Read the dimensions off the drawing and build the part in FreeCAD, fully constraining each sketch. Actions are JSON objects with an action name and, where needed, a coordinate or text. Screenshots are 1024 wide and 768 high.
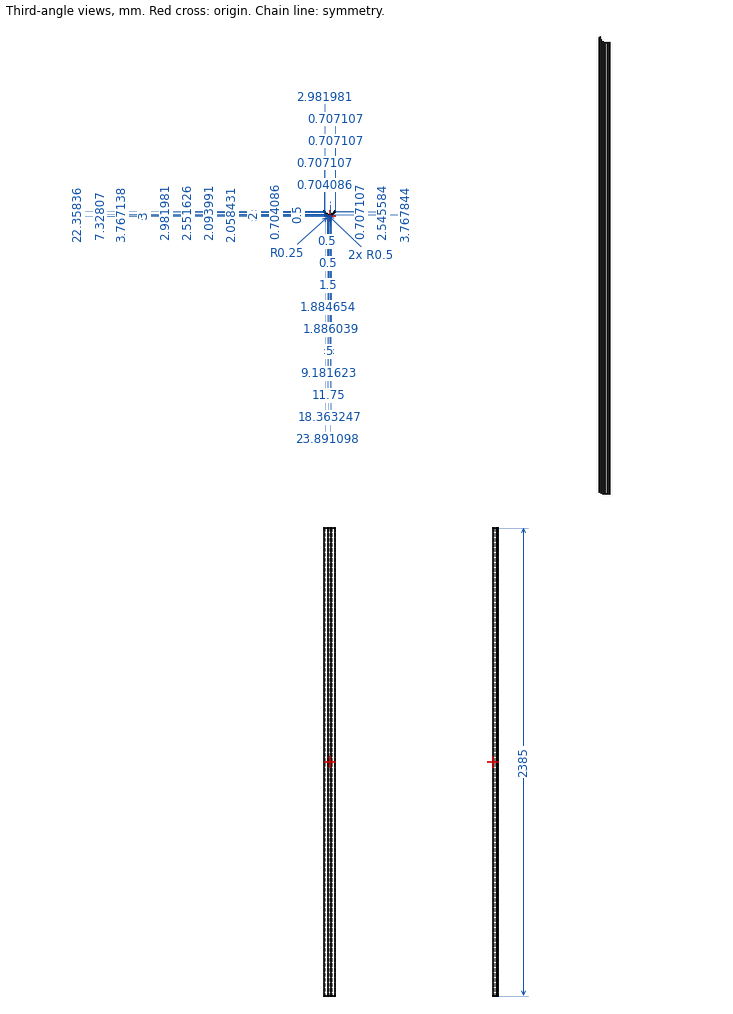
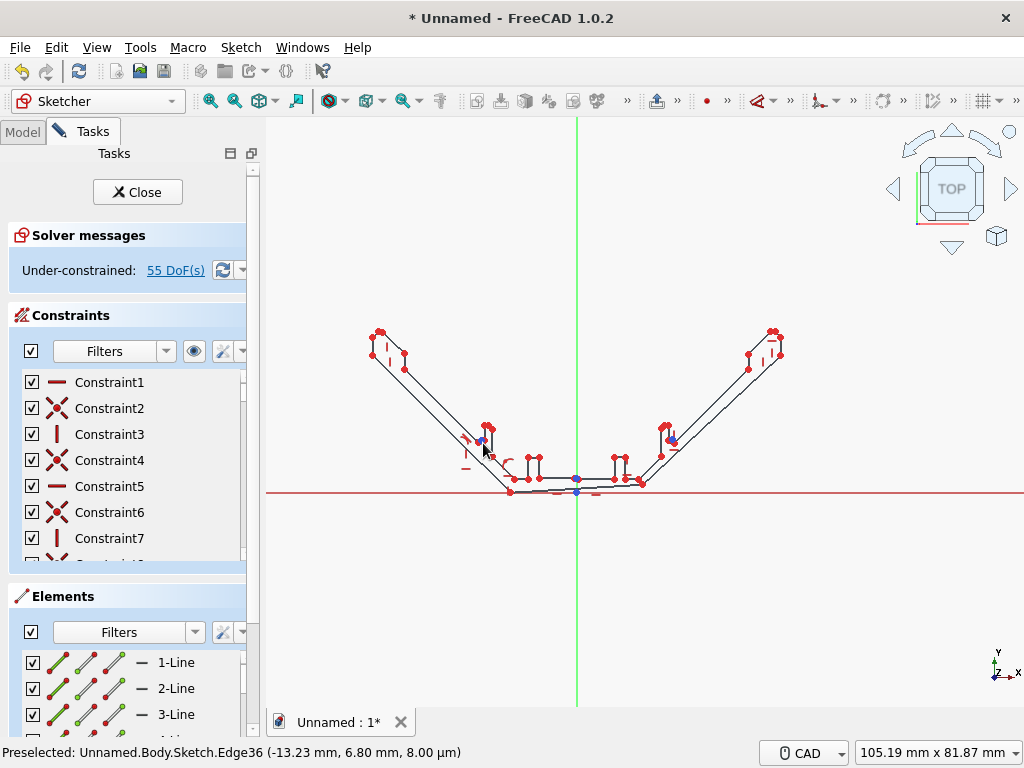
{"action": "scroll", "coordinate": [727, 391], "scroll_direction": "up", "scroll_amount": 2}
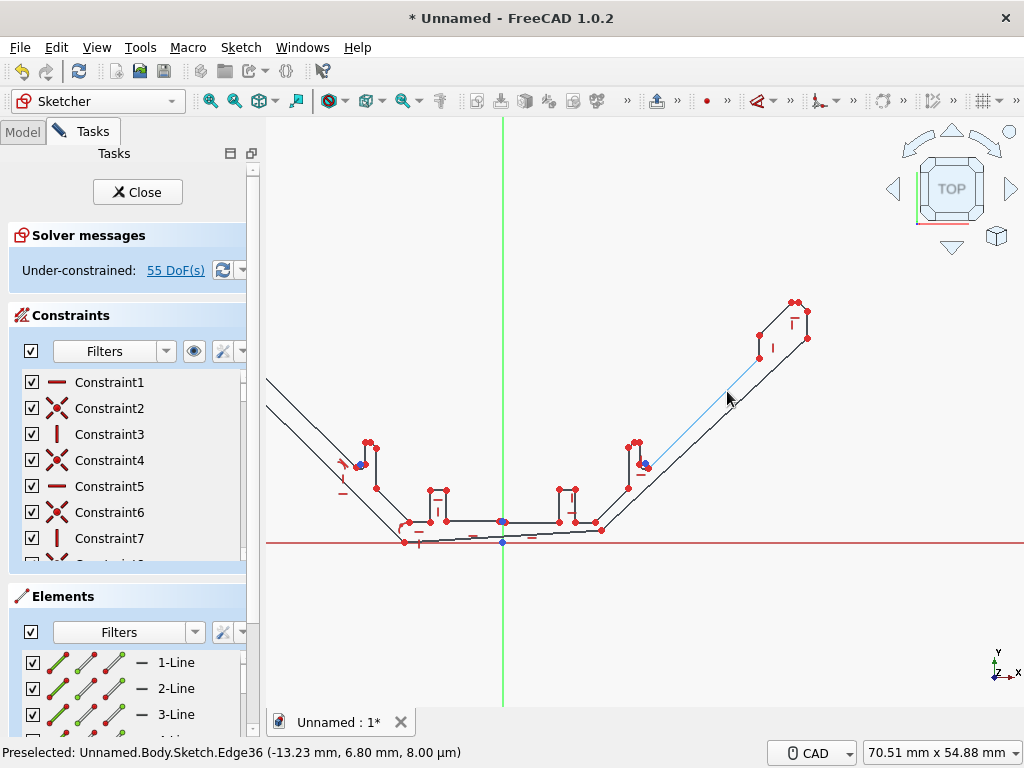
{"action": "left_click", "coordinate": [726, 391]}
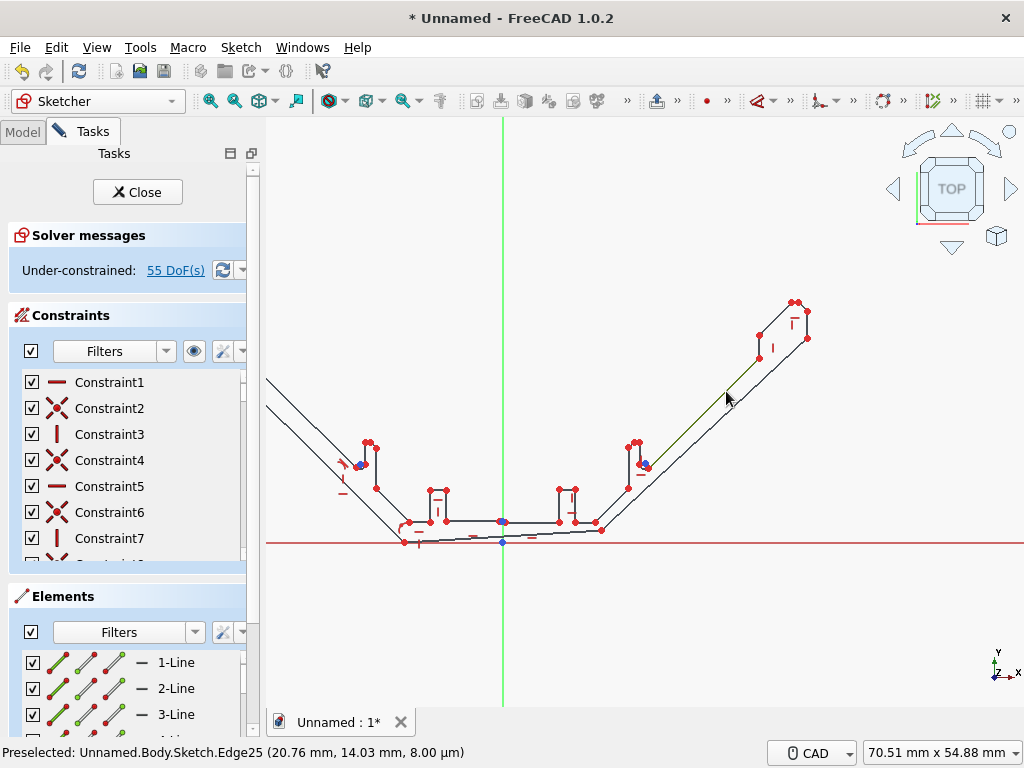
{"action": "scroll", "coordinate": [643, 469], "scroll_direction": "up", "scroll_amount": 5}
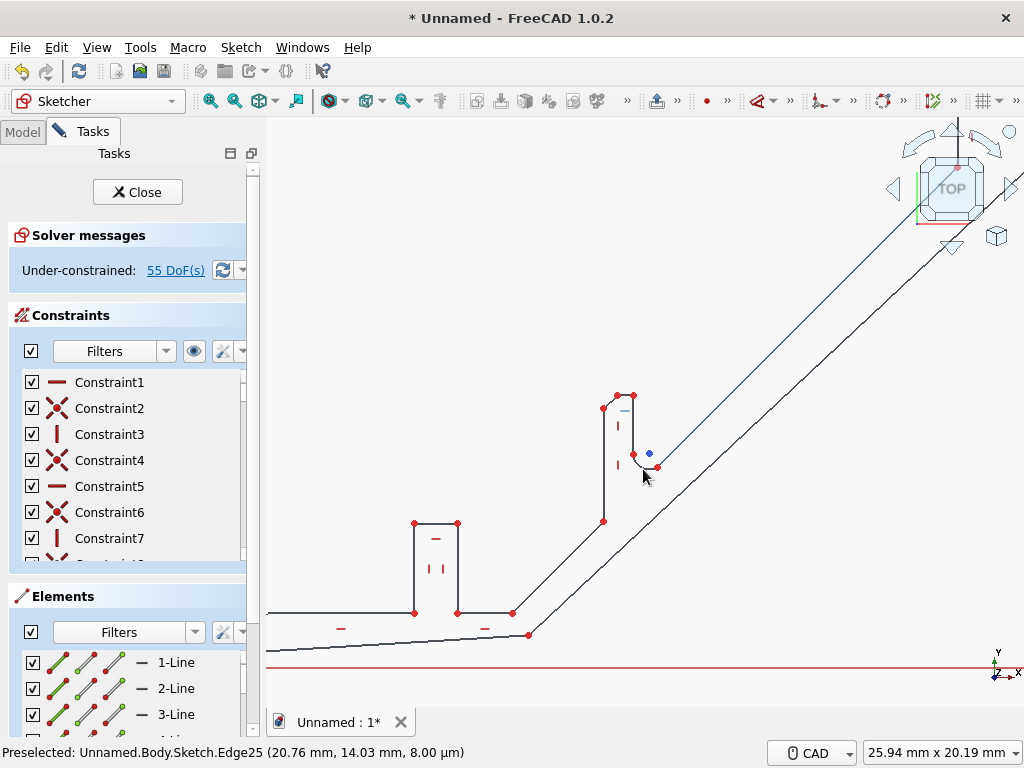
{"action": "left_click", "coordinate": [642, 468]}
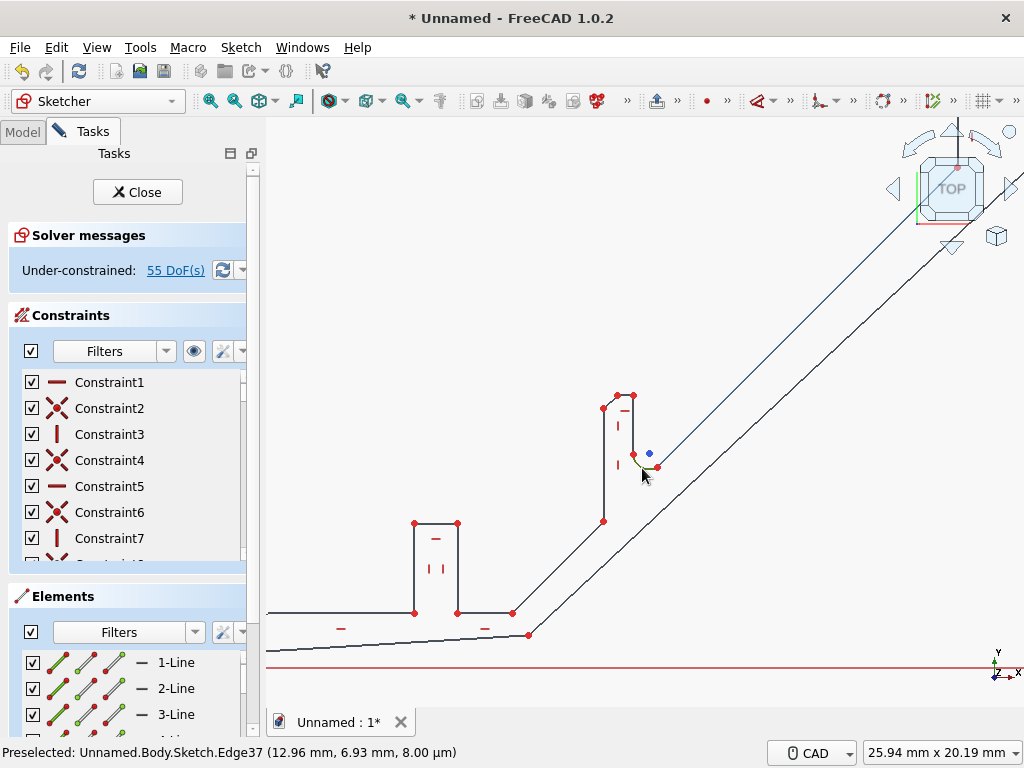
{"action": "key", "text": "t"}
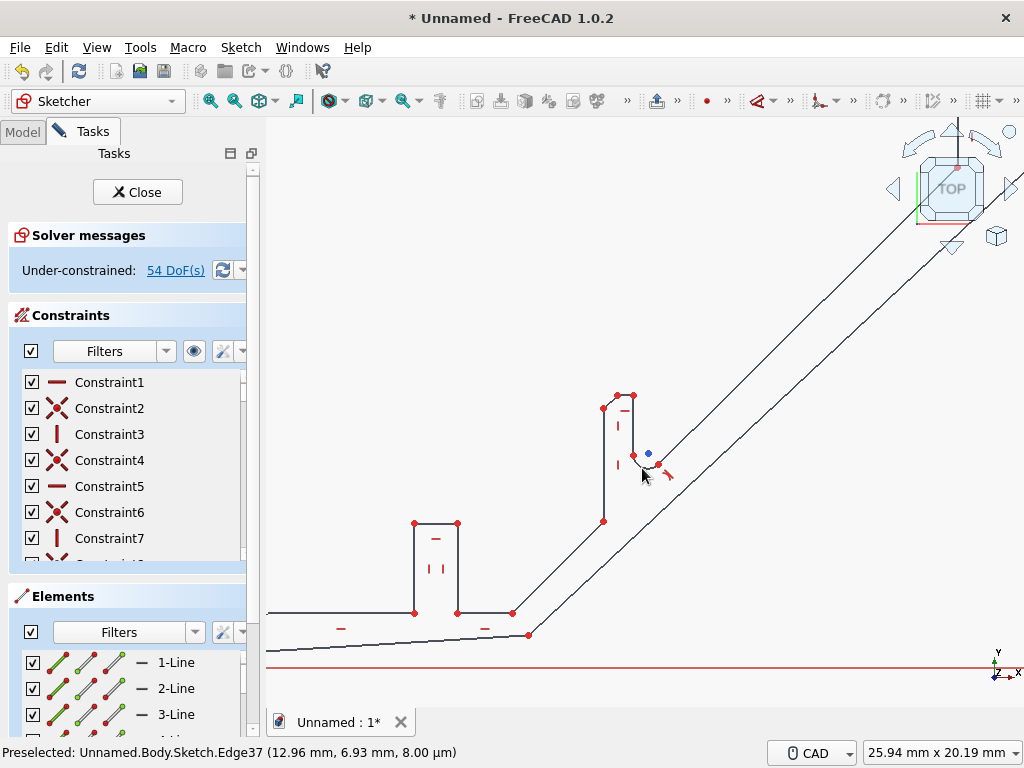
{"action": "left_click", "coordinate": [633, 437]}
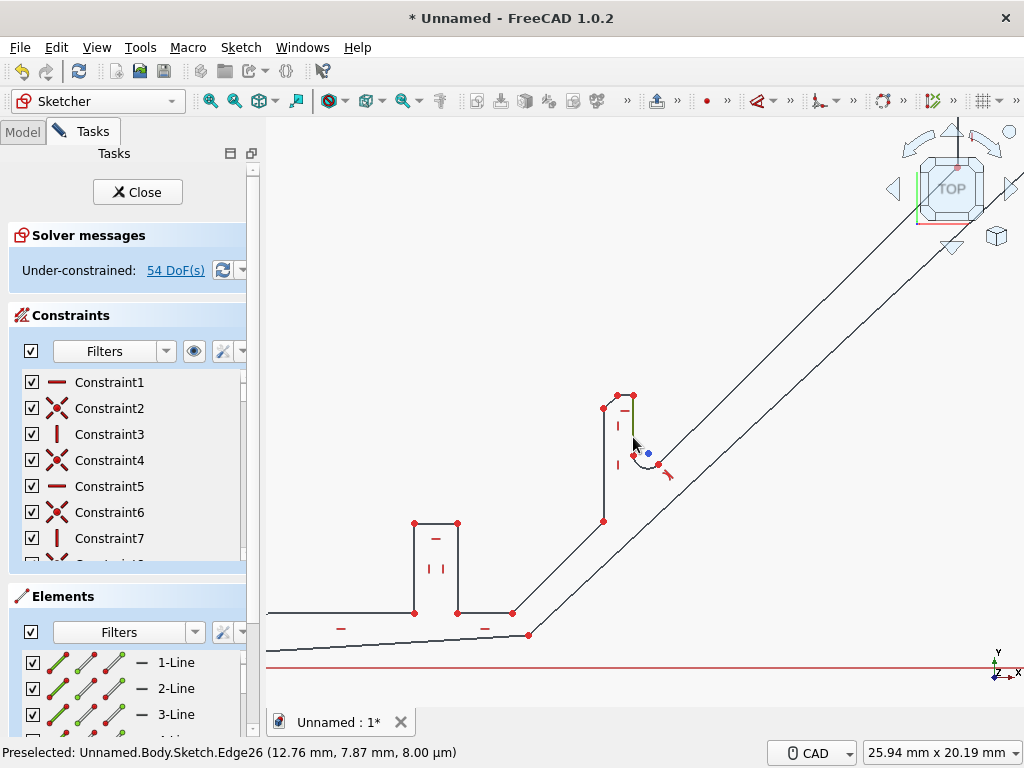
{"action": "scroll", "coordinate": [638, 464], "scroll_direction": "up", "scroll_amount": 2}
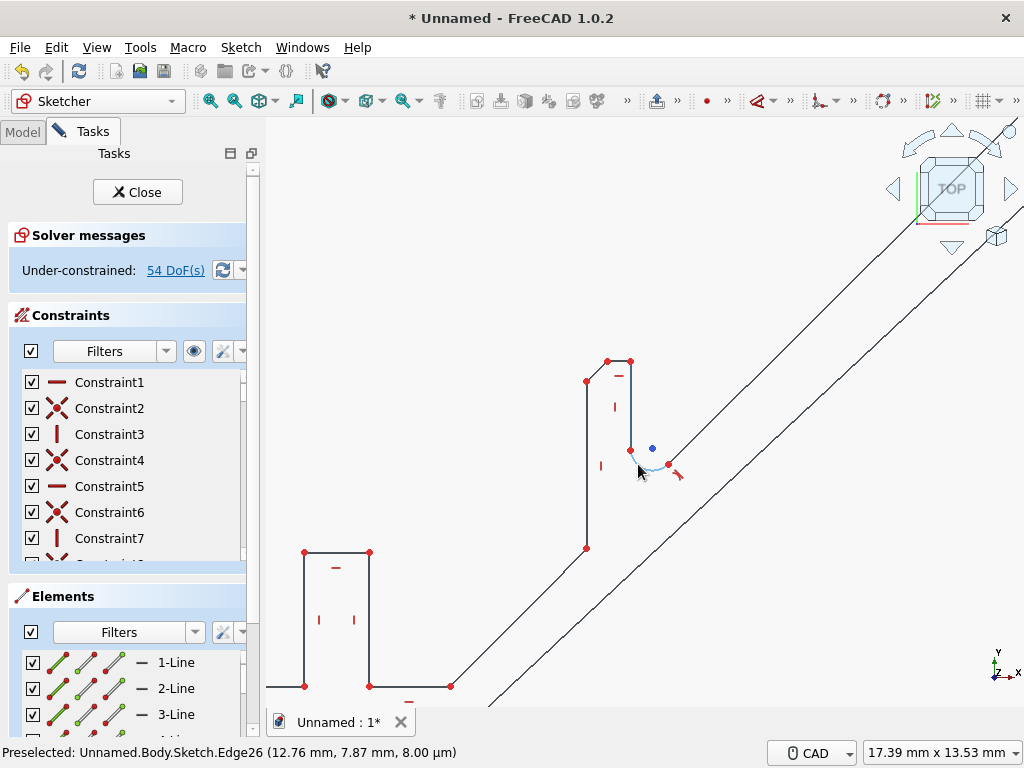
{"action": "left_click", "coordinate": [637, 464]}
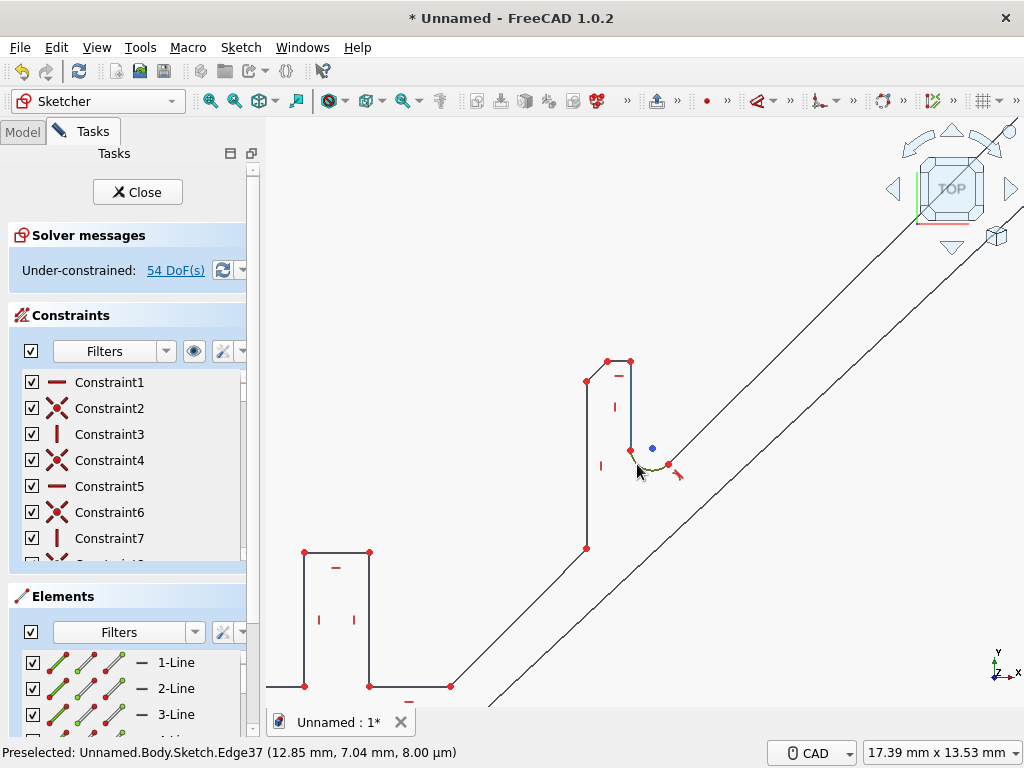
{"action": "key", "text": "t"}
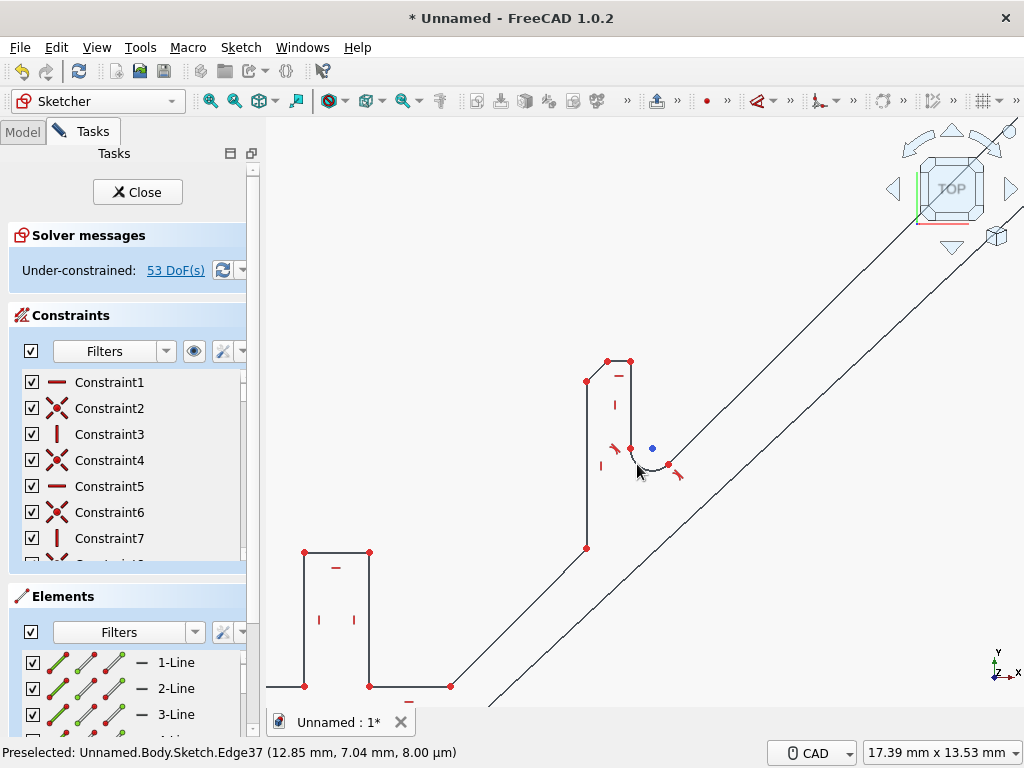
{"action": "scroll", "coordinate": [676, 438], "scroll_direction": "down", "scroll_amount": 9}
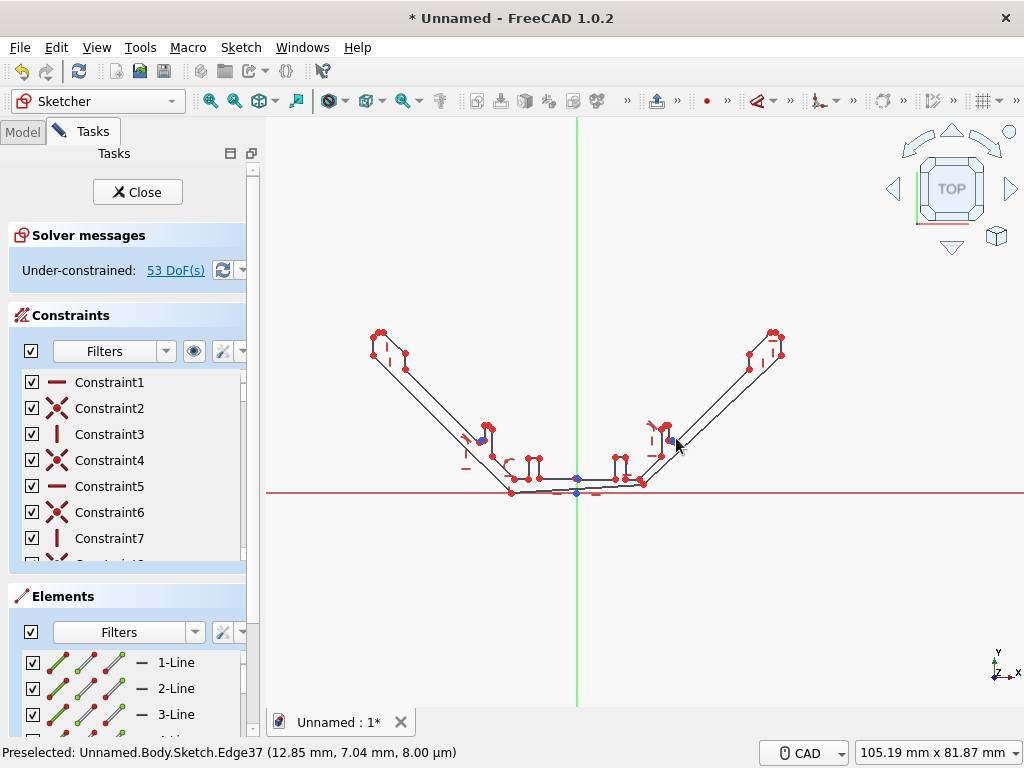
{"action": "scroll", "coordinate": [381, 333], "scroll_direction": "up", "scroll_amount": 10}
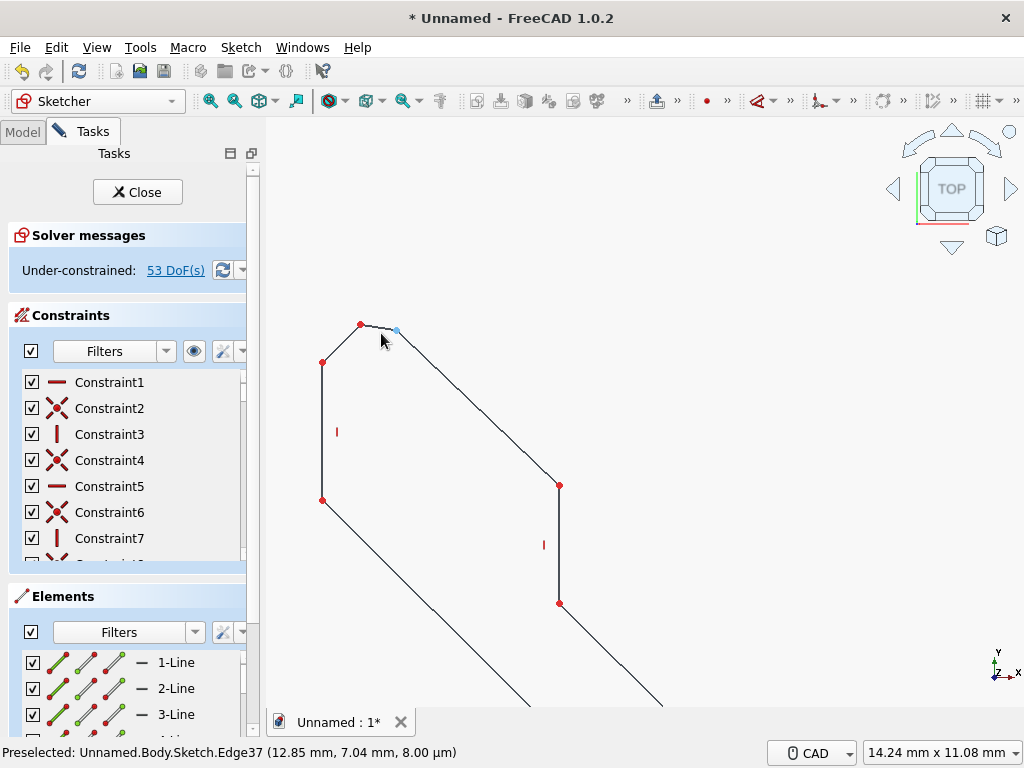
{"action": "left_click", "coordinate": [382, 328]}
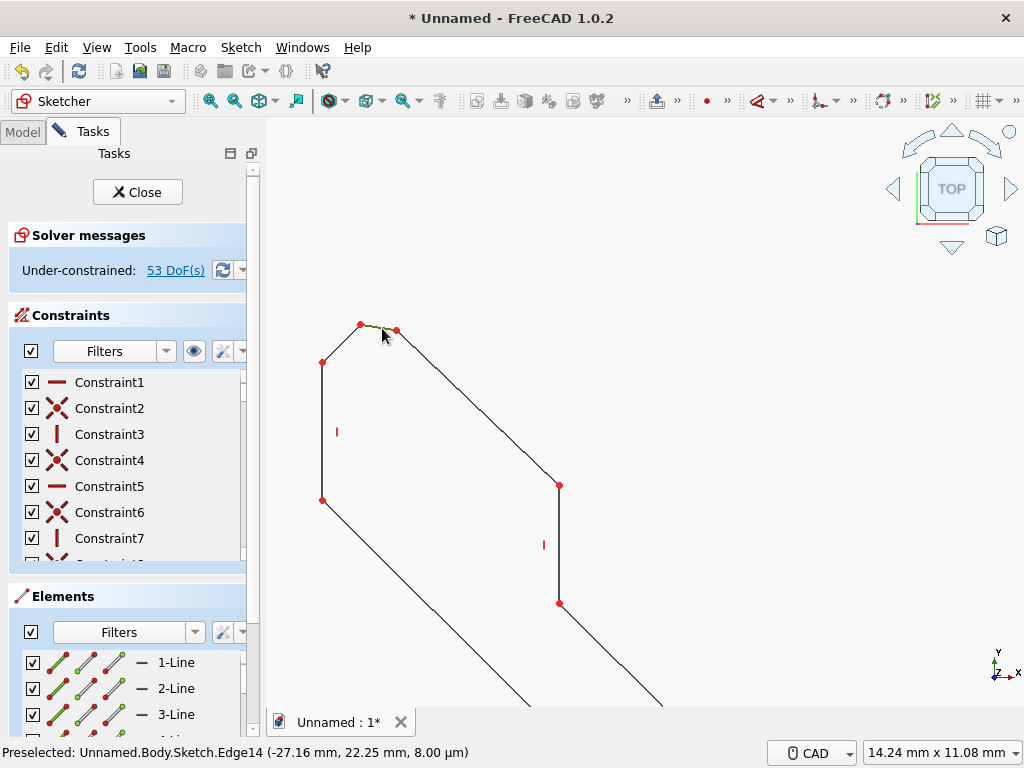
{"action": "key", "text": "h"}